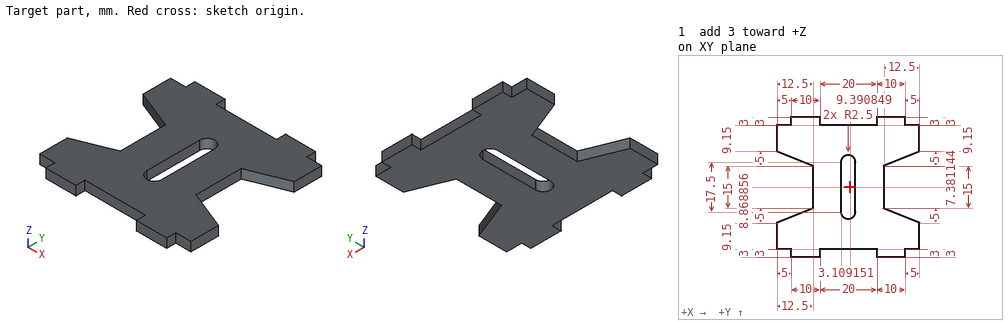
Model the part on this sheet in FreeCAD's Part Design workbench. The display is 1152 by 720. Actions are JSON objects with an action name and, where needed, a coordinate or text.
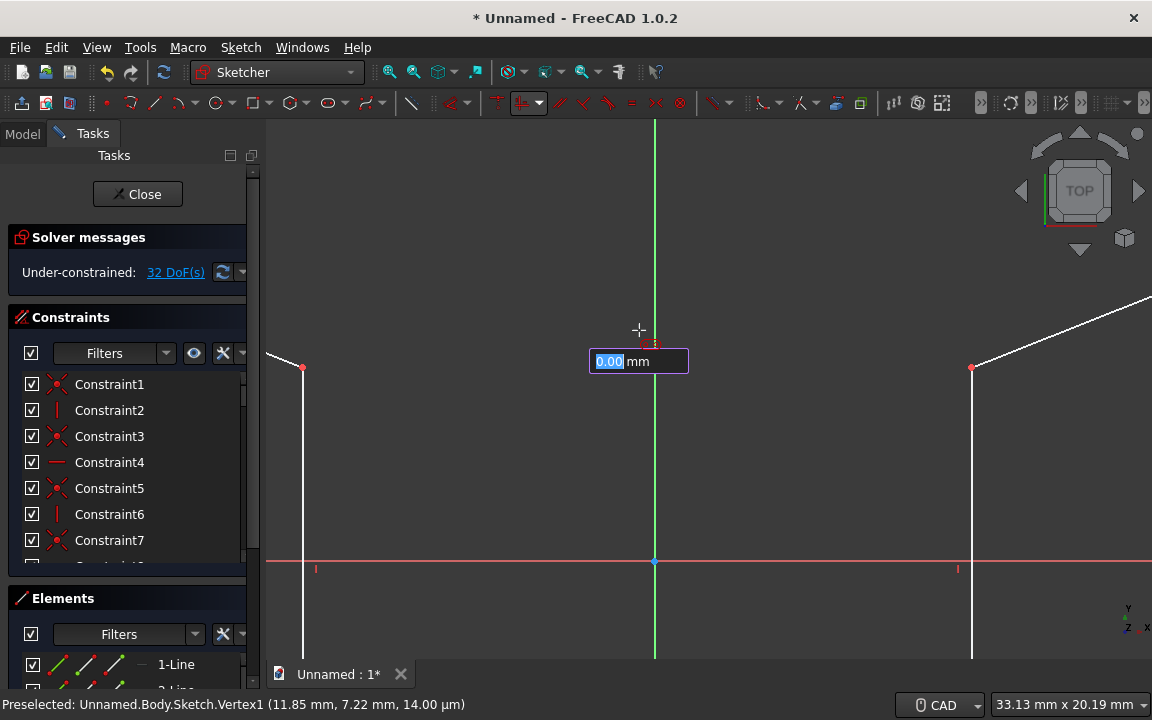
{"action": "scroll", "coordinate": [641, 332], "scroll_direction": "down", "scroll_amount": 7}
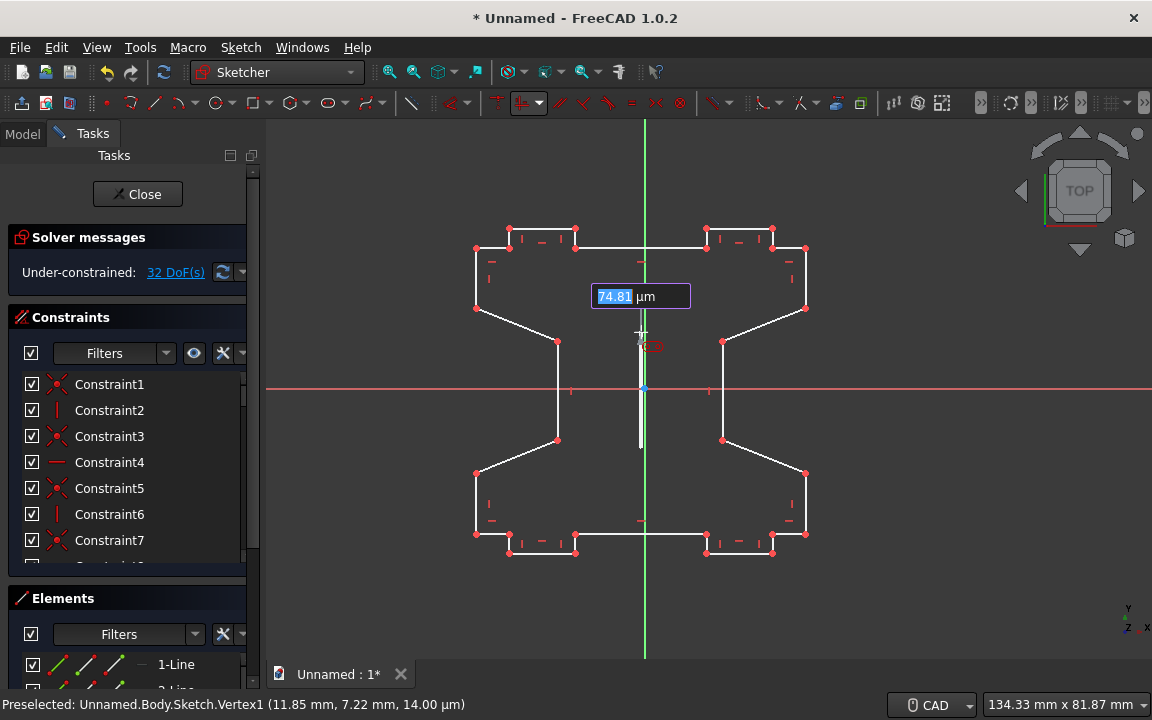
{"action": "scroll", "coordinate": [657, 372], "scroll_direction": "up", "scroll_amount": 2}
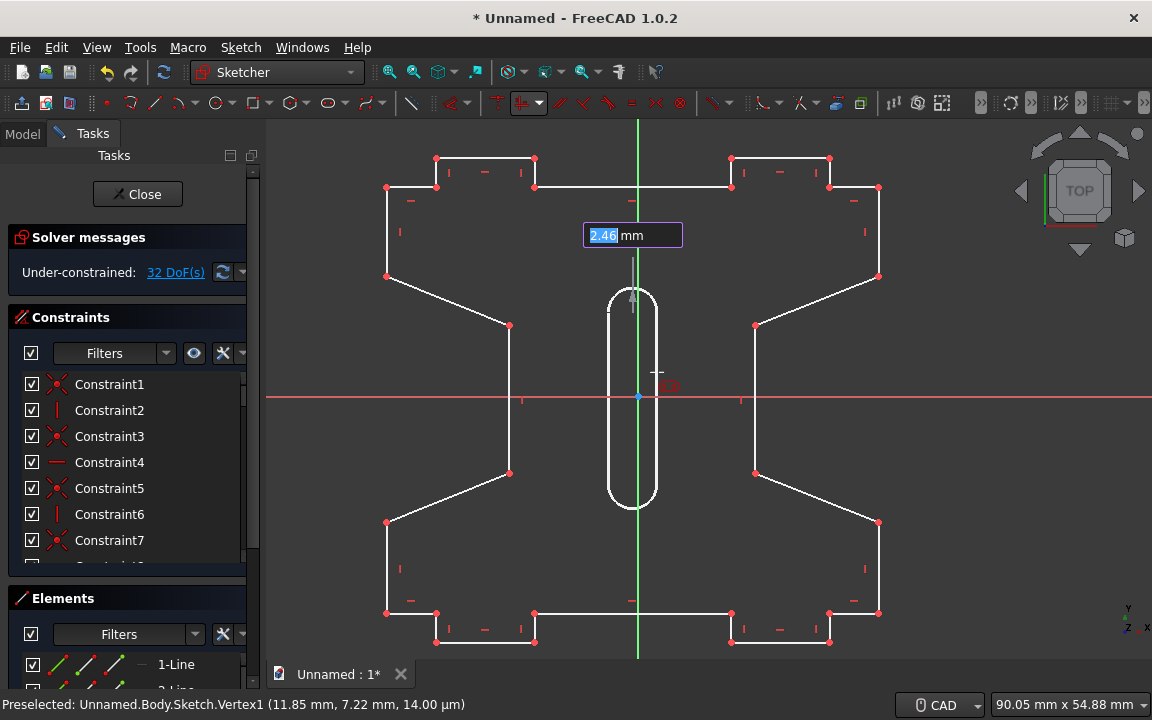
{"action": "left_click", "coordinate": [657, 372]}
{"action": "key", "text": "Escape"}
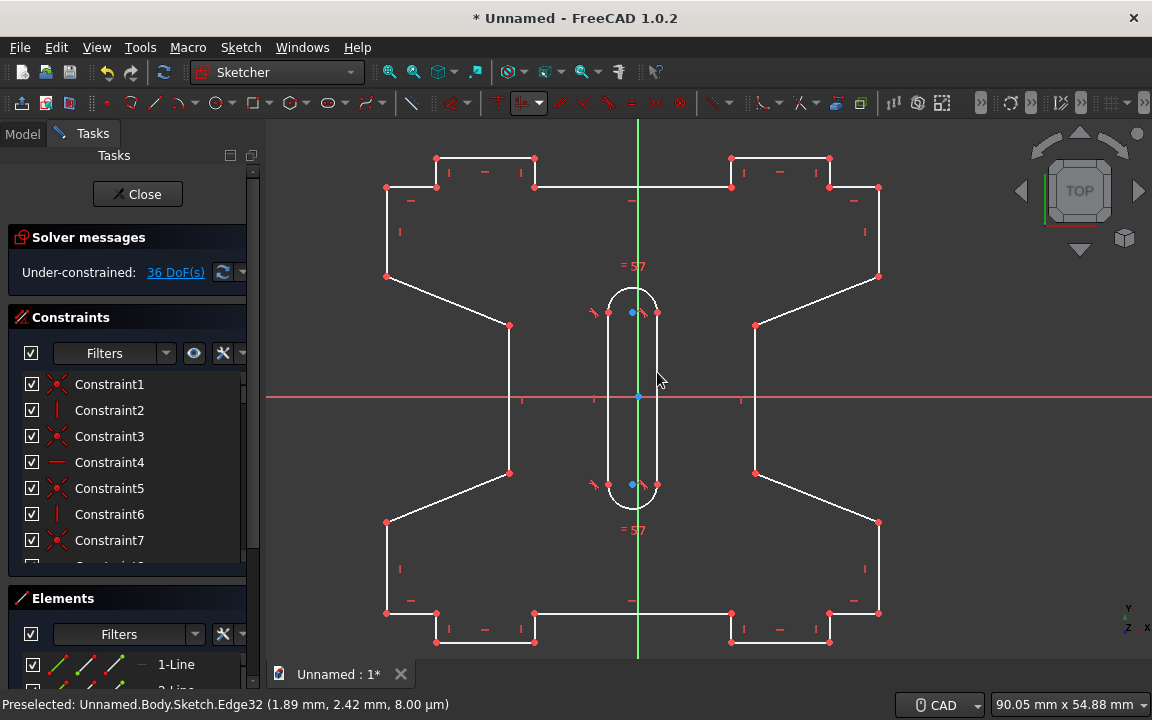
{"action": "scroll", "coordinate": [618, 504], "scroll_direction": "up", "scroll_amount": 3}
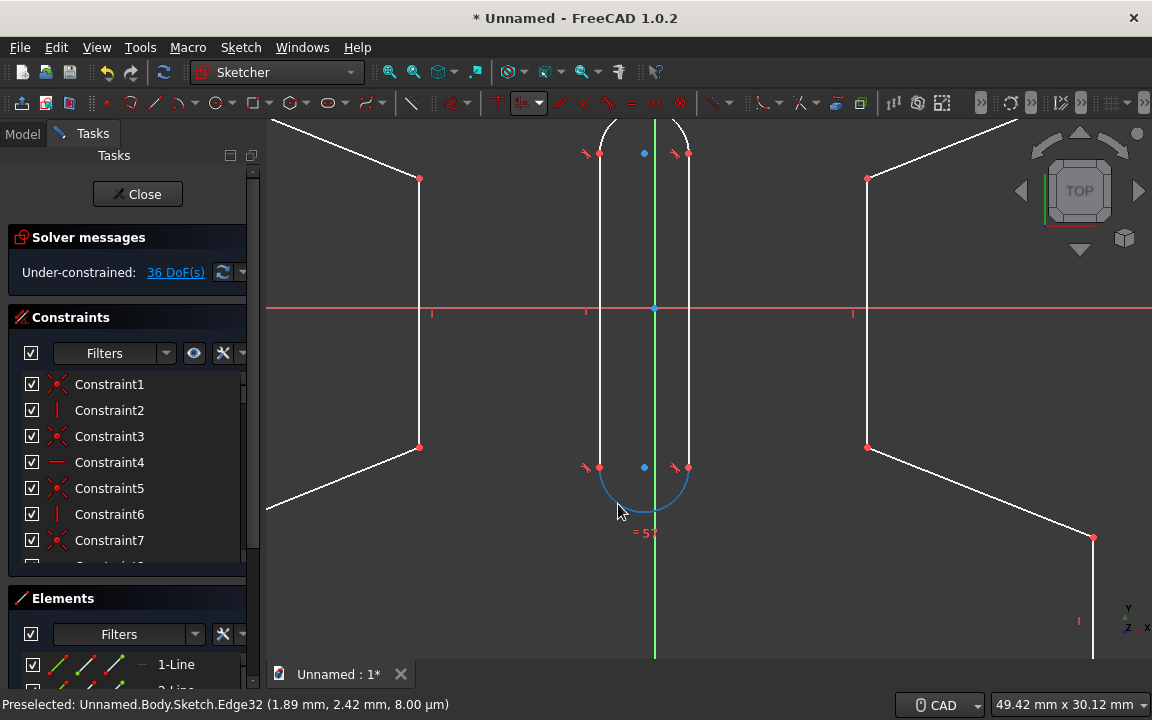
{"action": "left_click", "coordinate": [618, 504]}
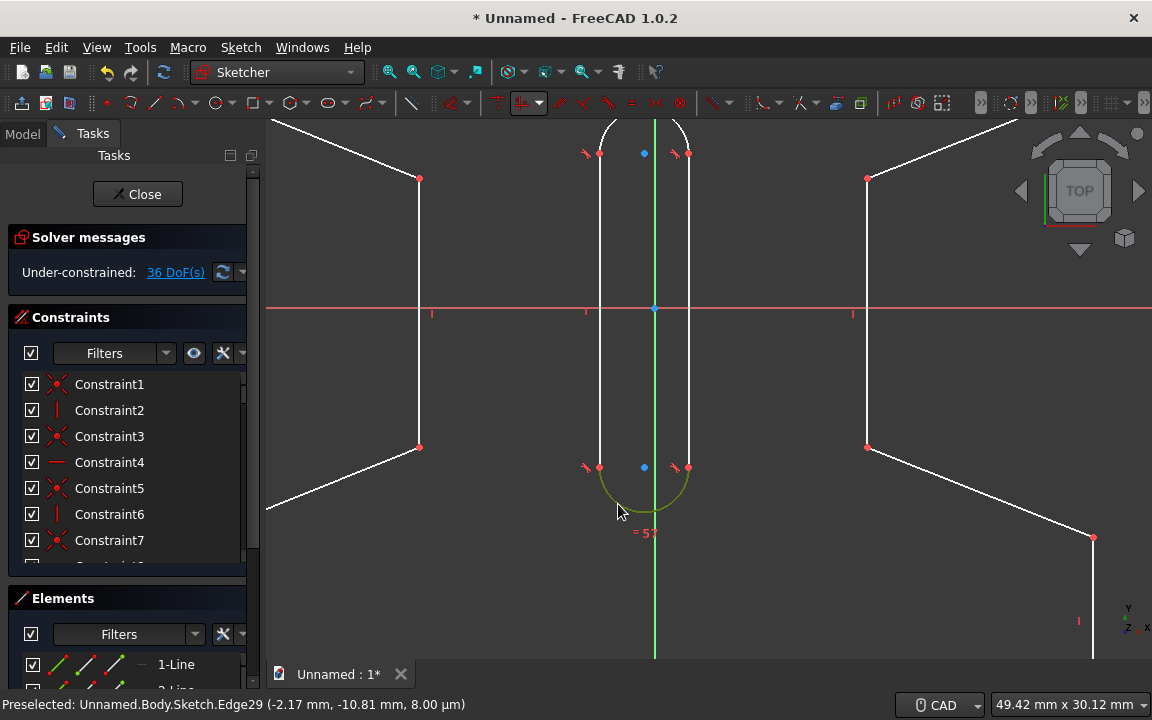
{"action": "key", "text": "k r"}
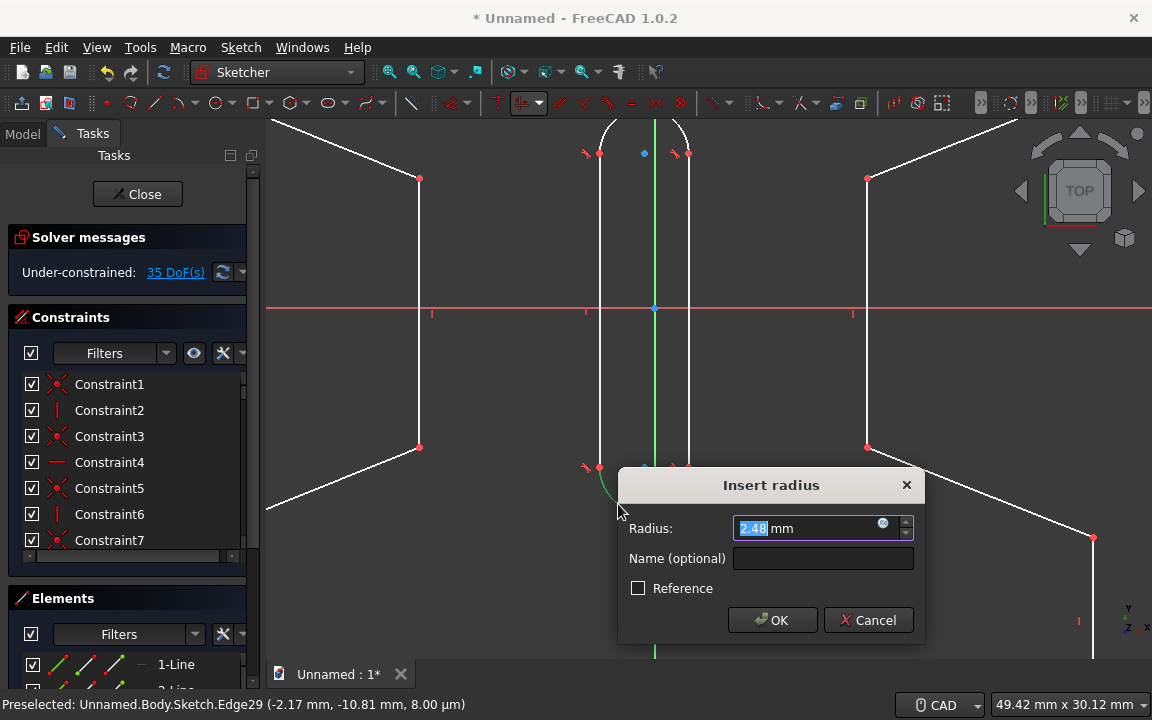
{"action": "type", "text": "2.5"}
{"action": "key", "text": "Return"}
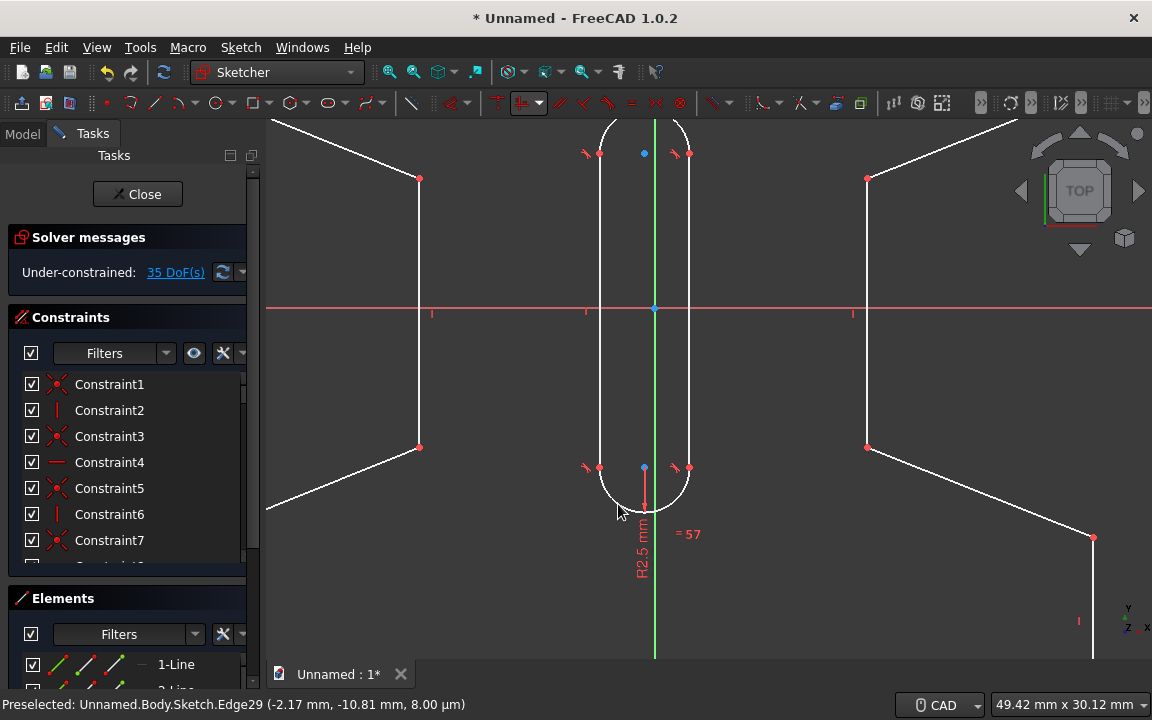
{"action": "scroll", "coordinate": [638, 435], "scroll_direction": "down", "scroll_amount": 5}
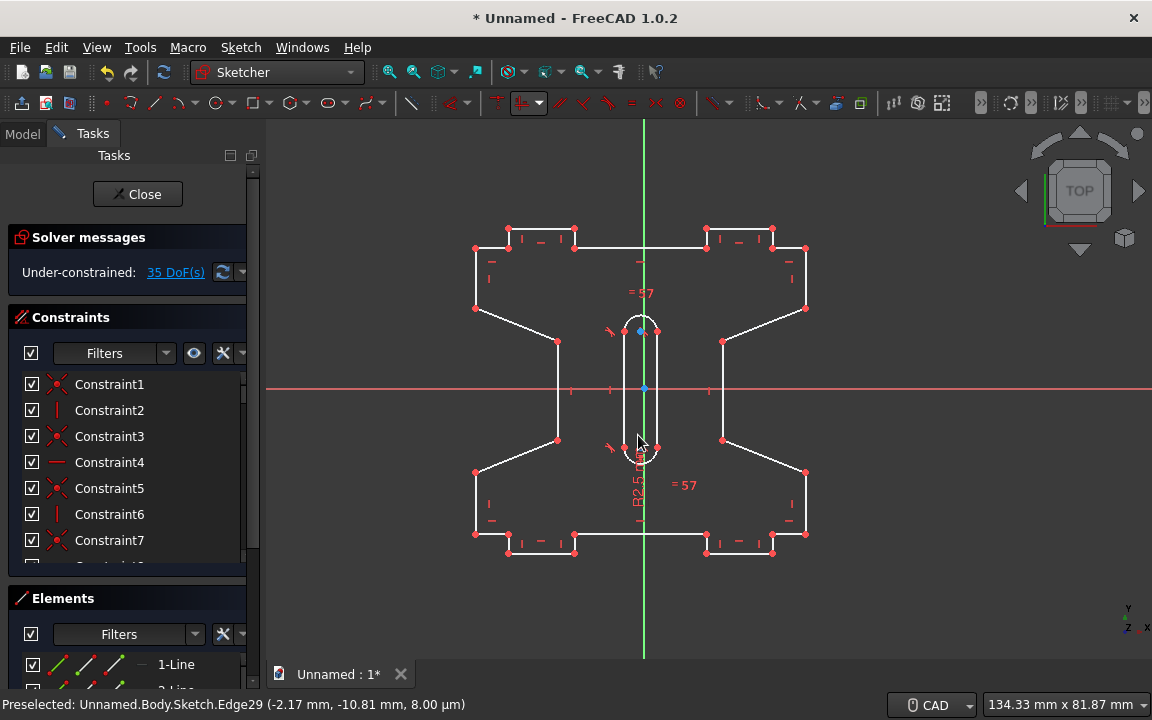
{"action": "scroll", "coordinate": [796, 248], "scroll_direction": "up", "scroll_amount": 2}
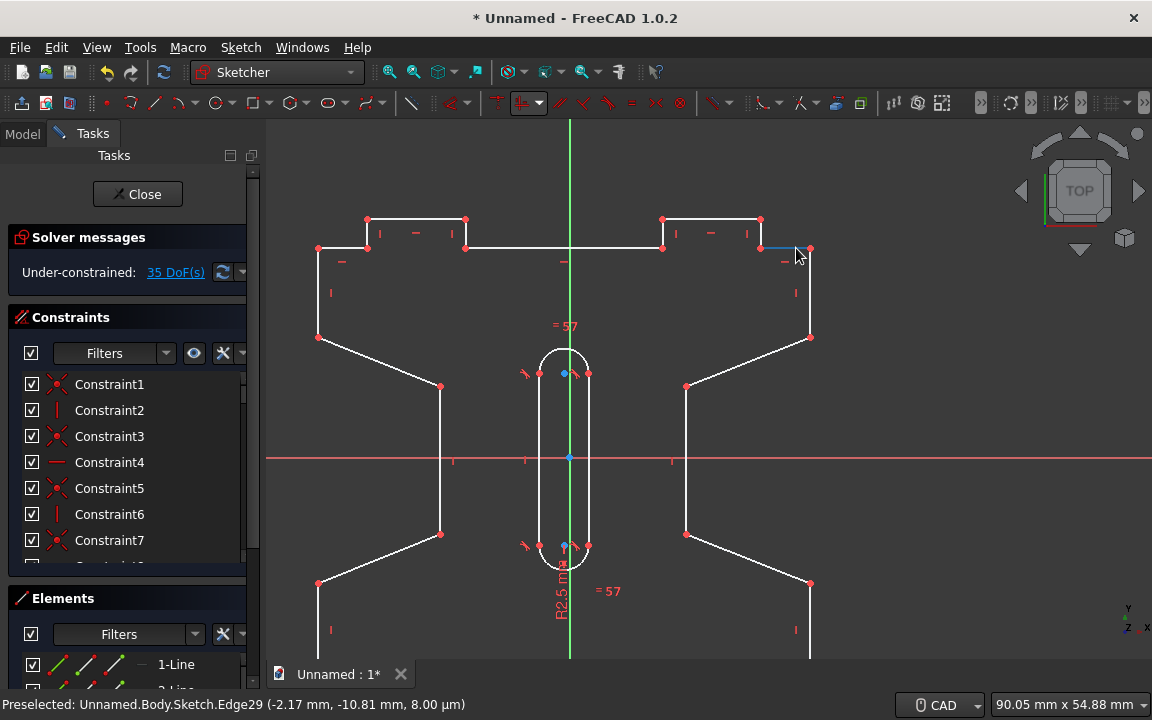
{"action": "left_click", "coordinate": [795, 248]}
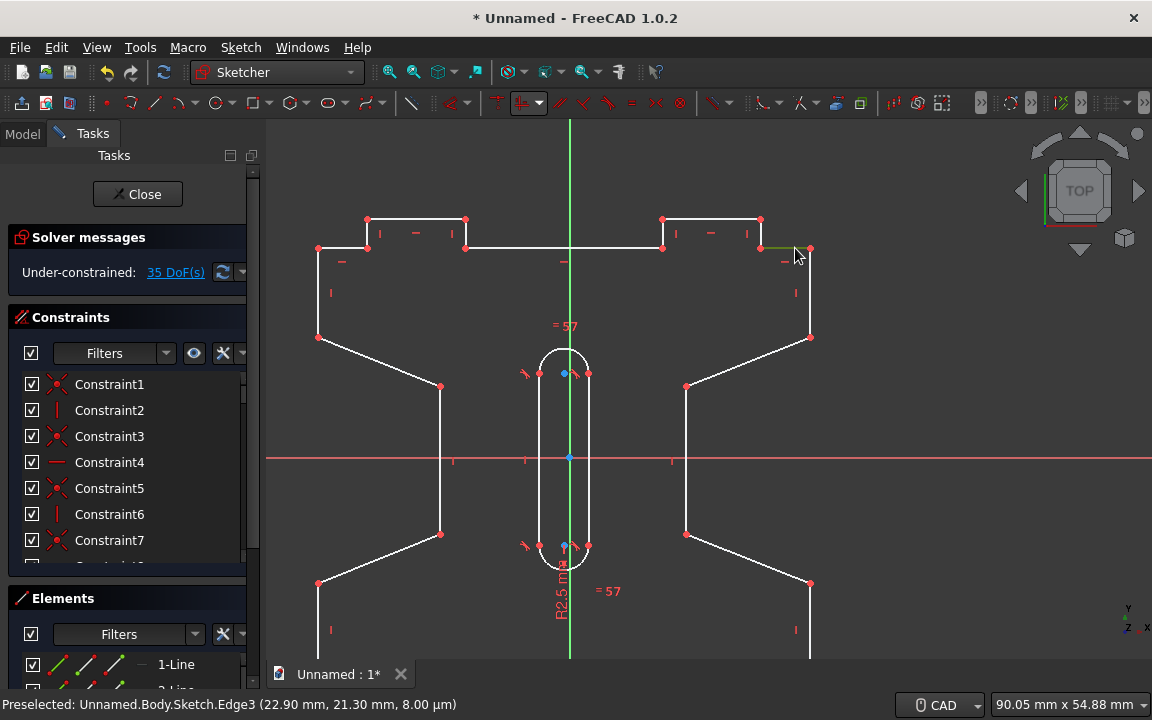
{"action": "left_click", "coordinate": [470, 104]}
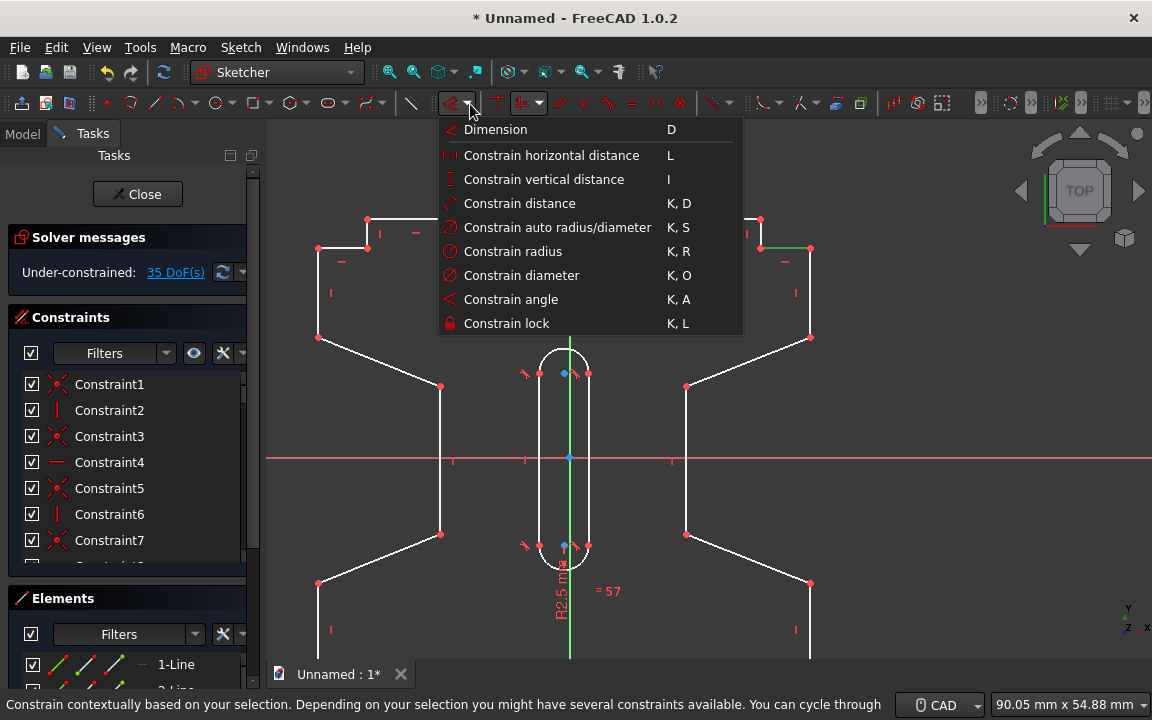
{"action": "left_click", "coordinate": [591, 155]}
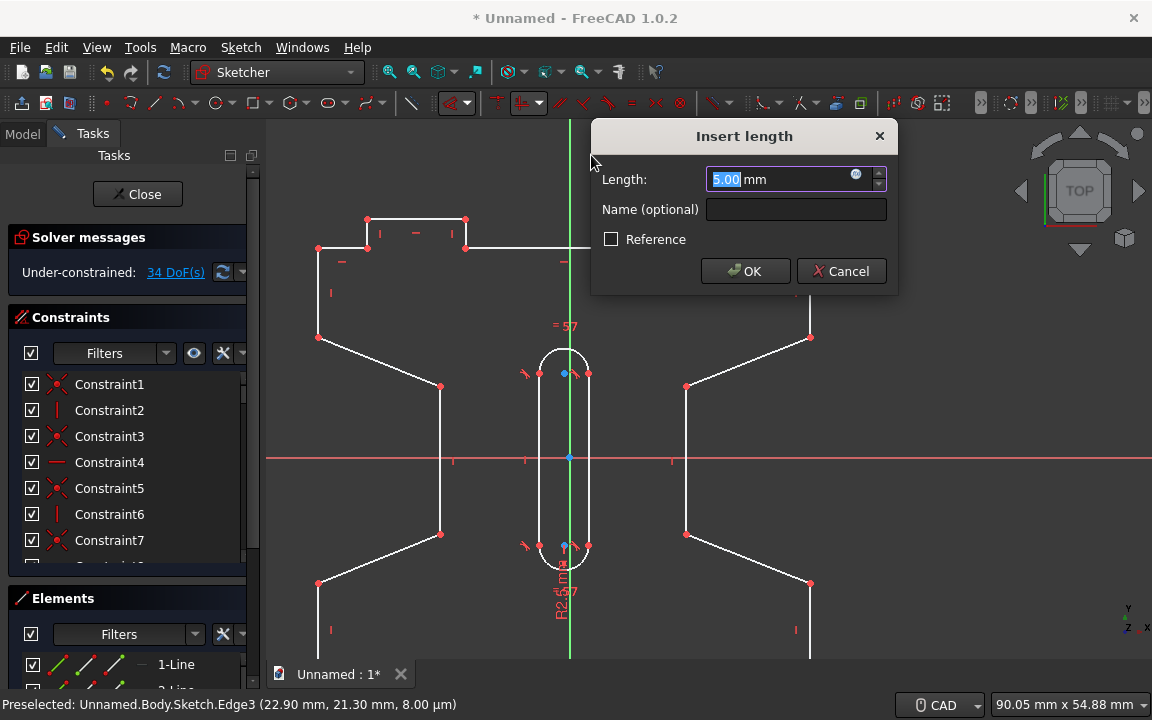
{"action": "type", "text": "5"}
{"action": "key", "text": "Return"}